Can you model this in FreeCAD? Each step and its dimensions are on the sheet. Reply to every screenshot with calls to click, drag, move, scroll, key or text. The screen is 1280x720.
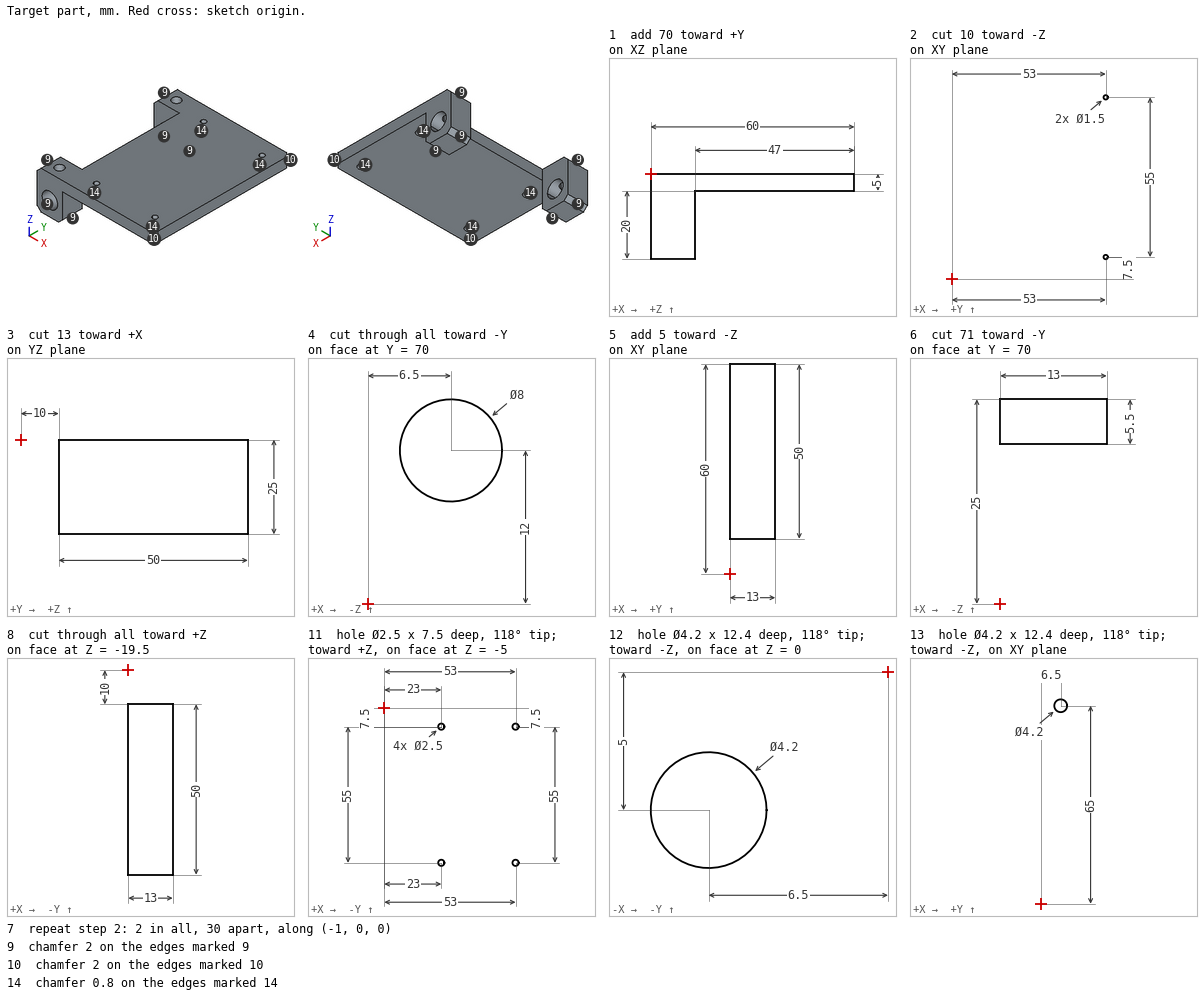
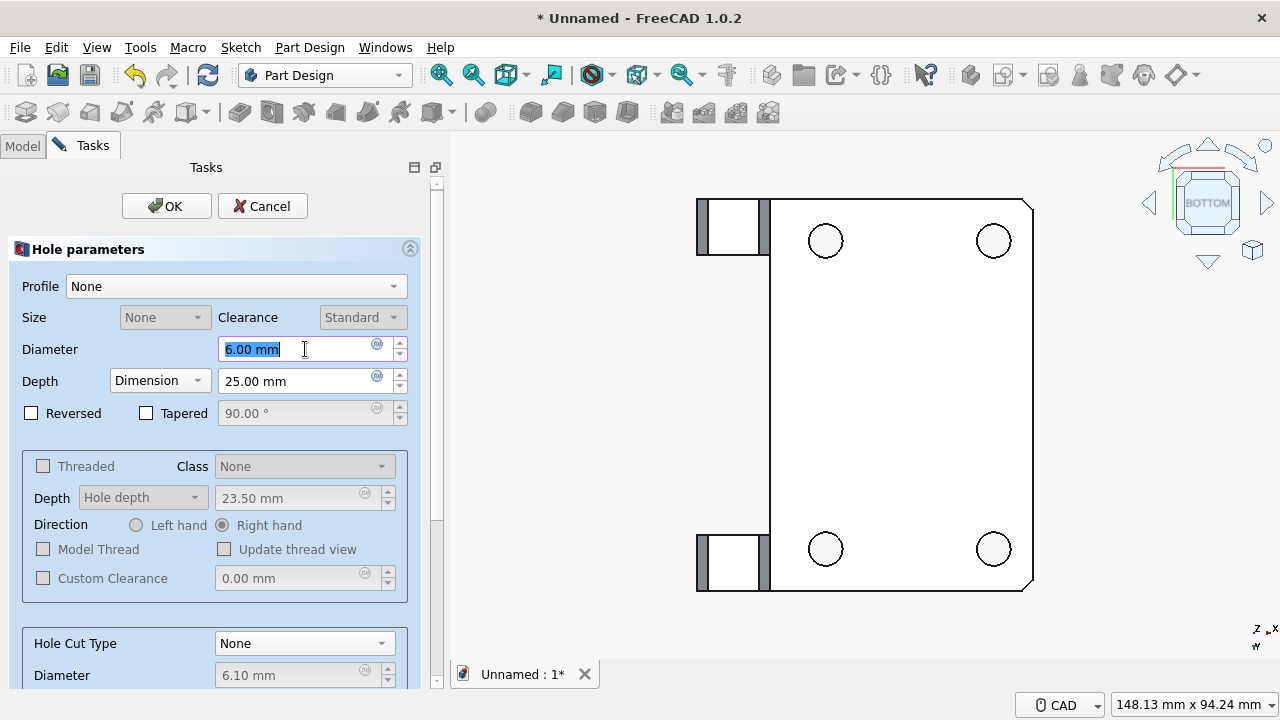
text(2.5)
key(Tab)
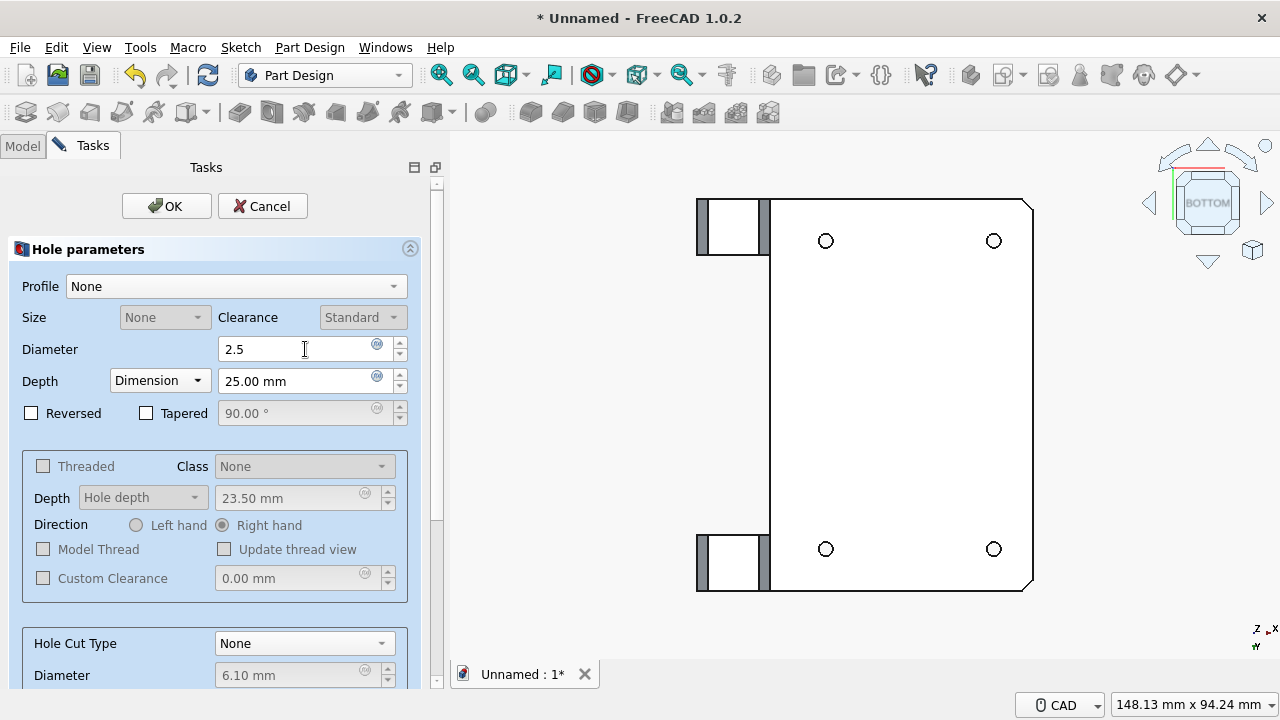
triple_click(305, 381)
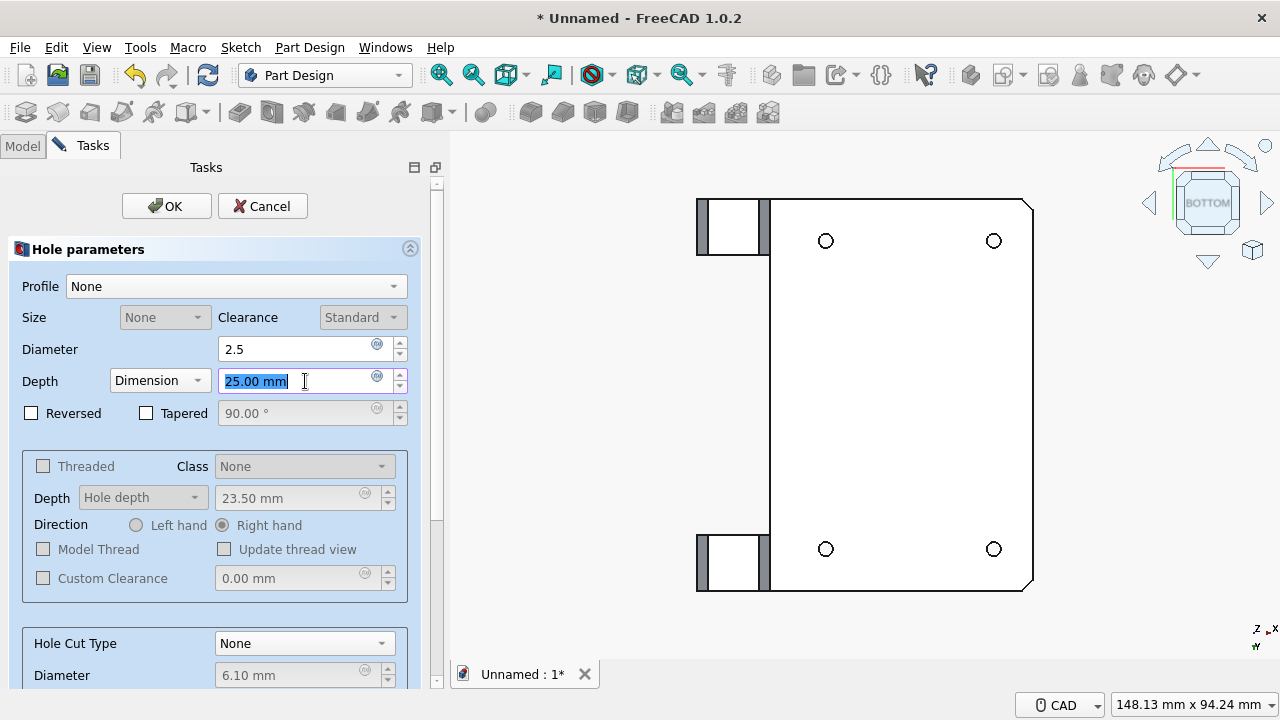
text(7.5)
key(Tab)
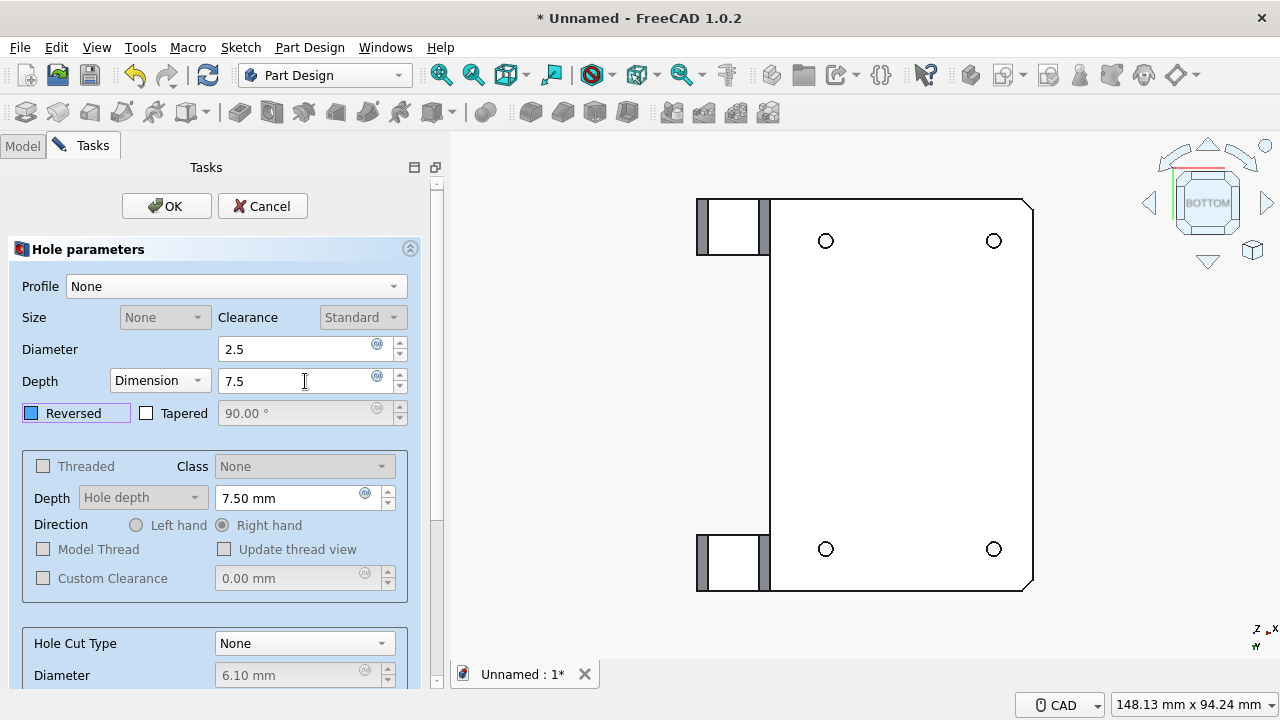
click(167, 206)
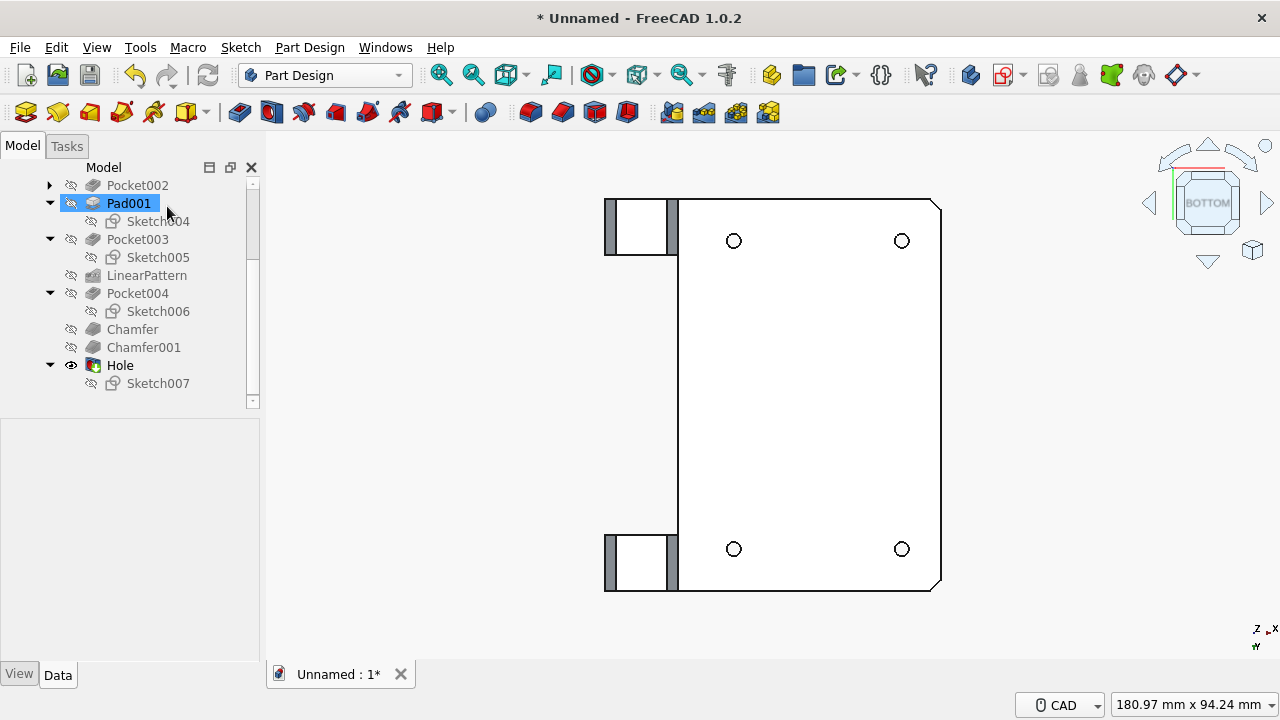
key(0)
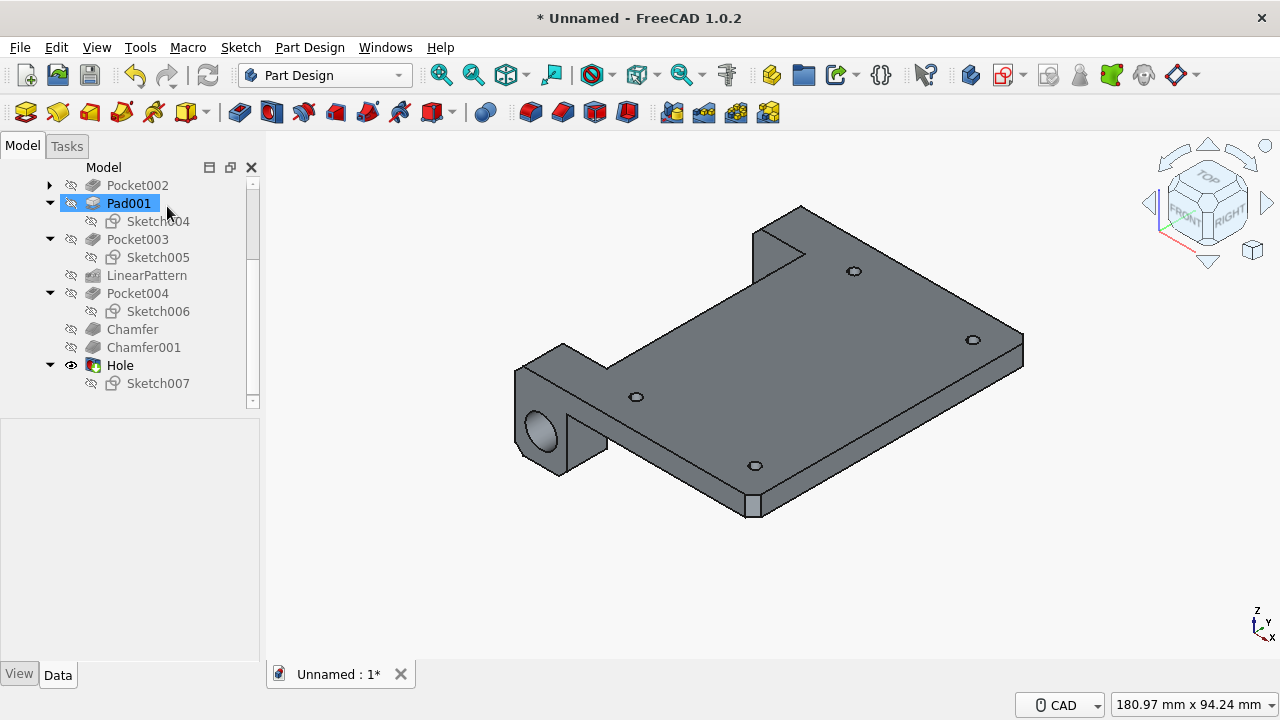
click(849, 348)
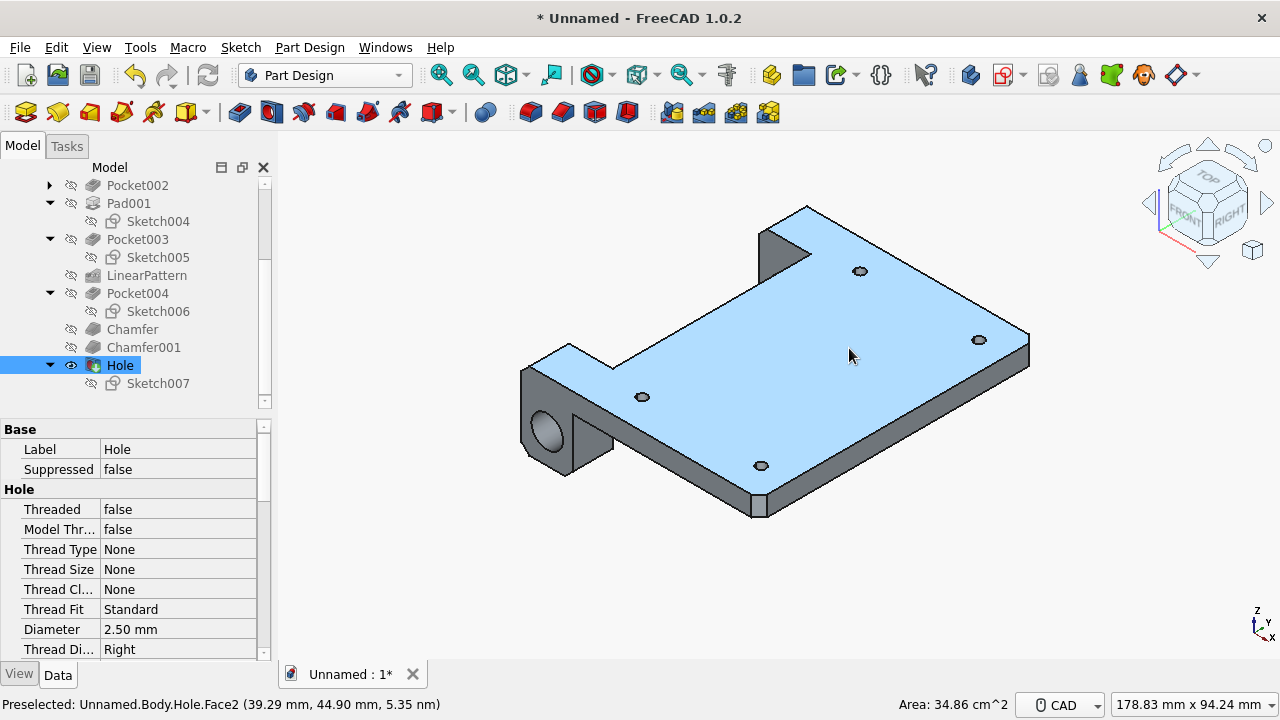
click(1004, 76)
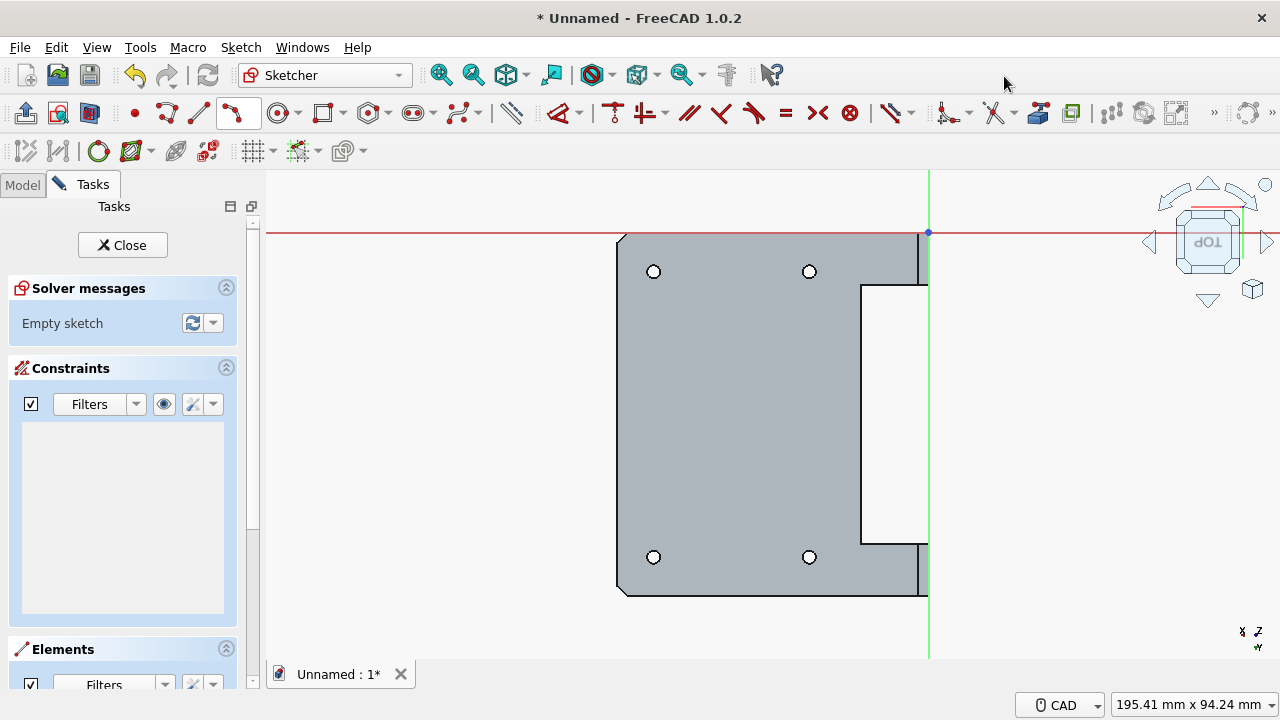
scroll(932, 231, up, 11)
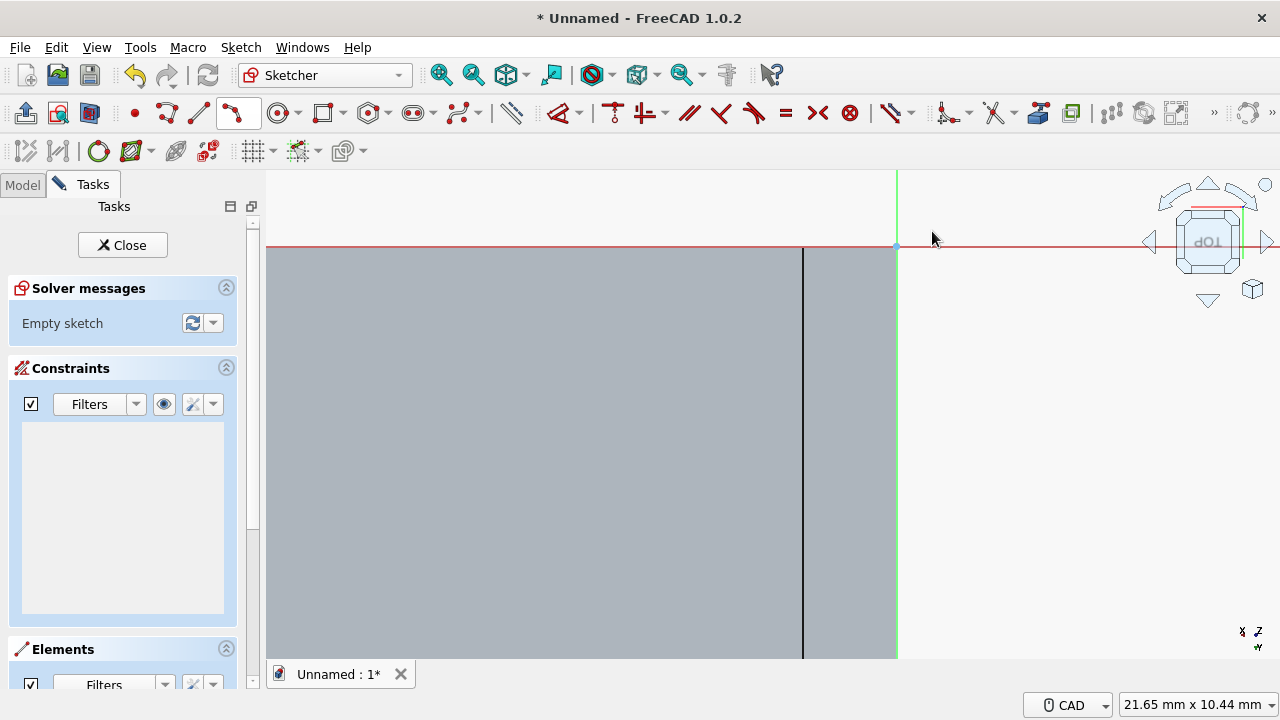
key(g)
key(c)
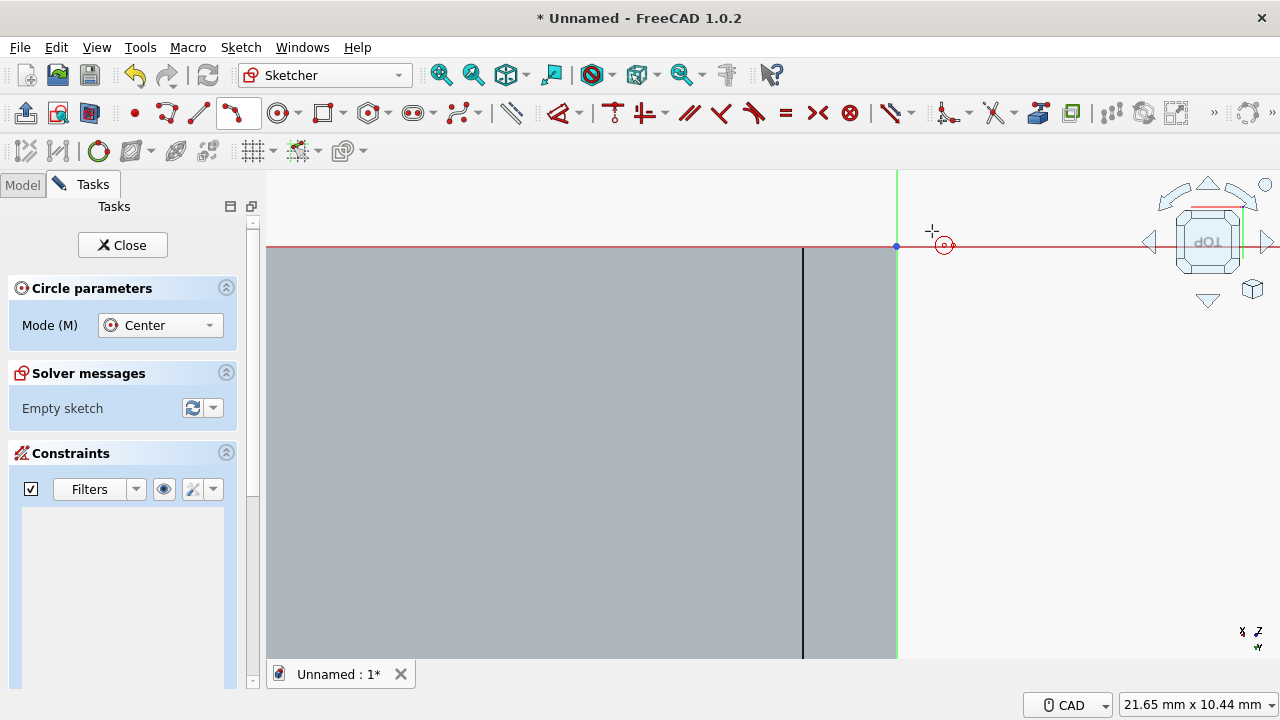
click(592, 481)
move(662, 412)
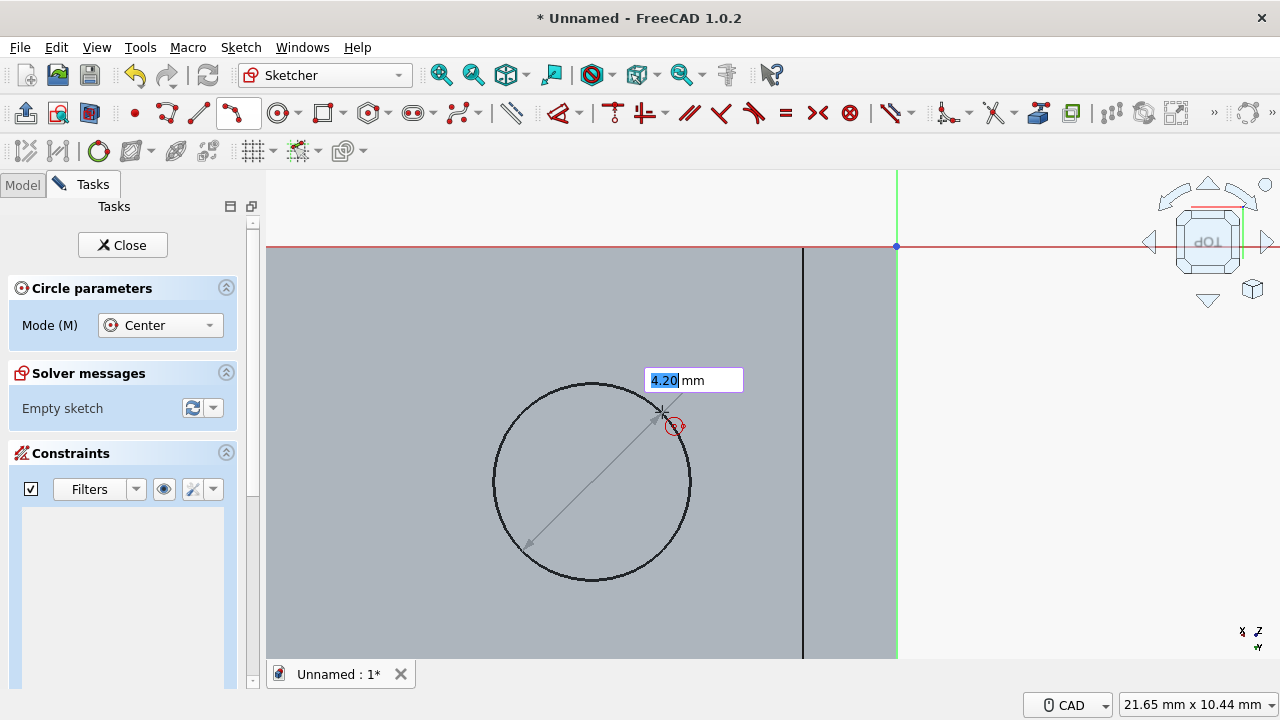
text(4.2)
key(Return)
key(Escape)